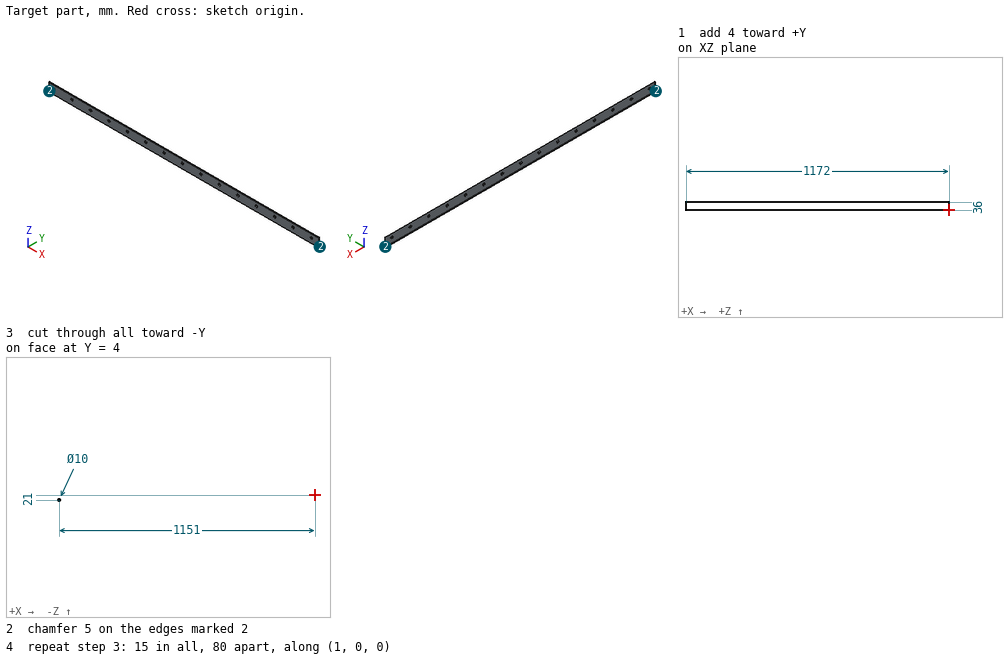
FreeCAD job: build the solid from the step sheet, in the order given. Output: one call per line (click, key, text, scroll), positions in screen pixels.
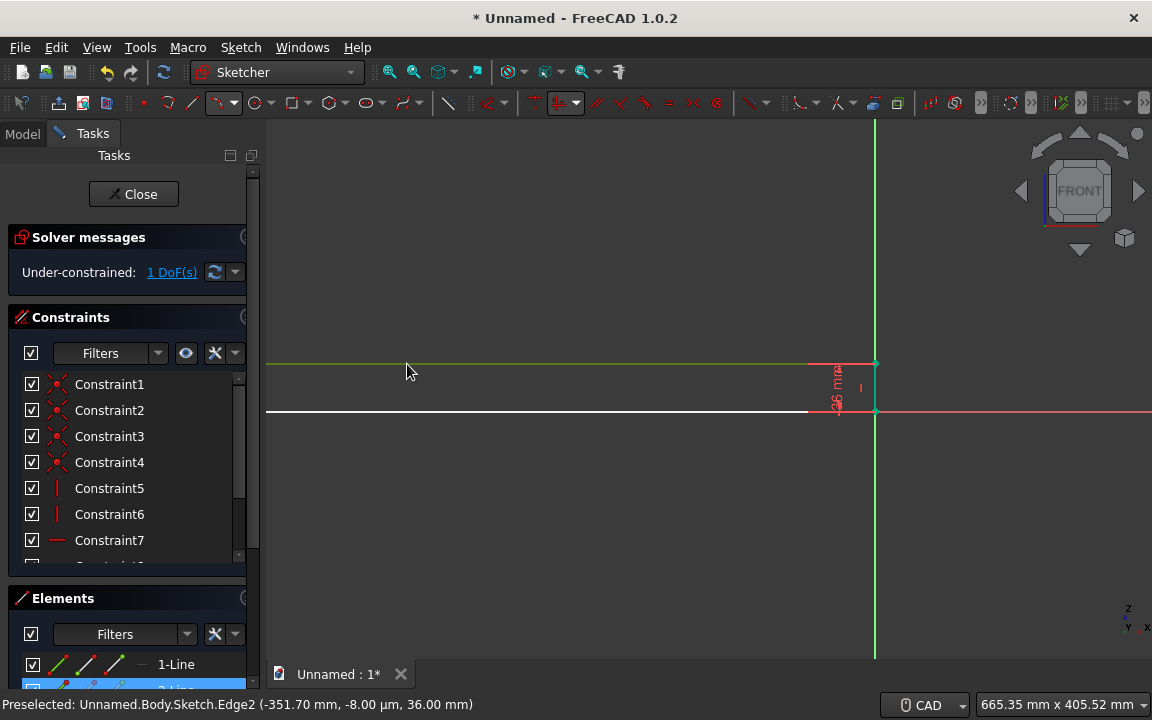
click(506, 104)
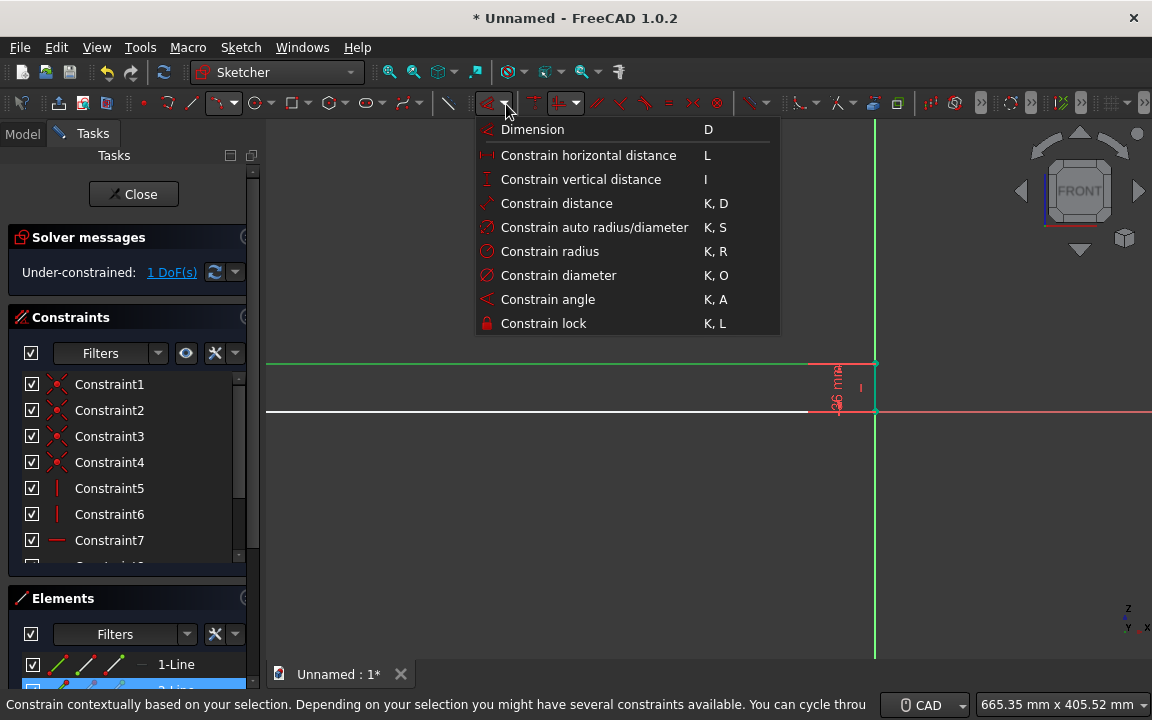
click(628, 155)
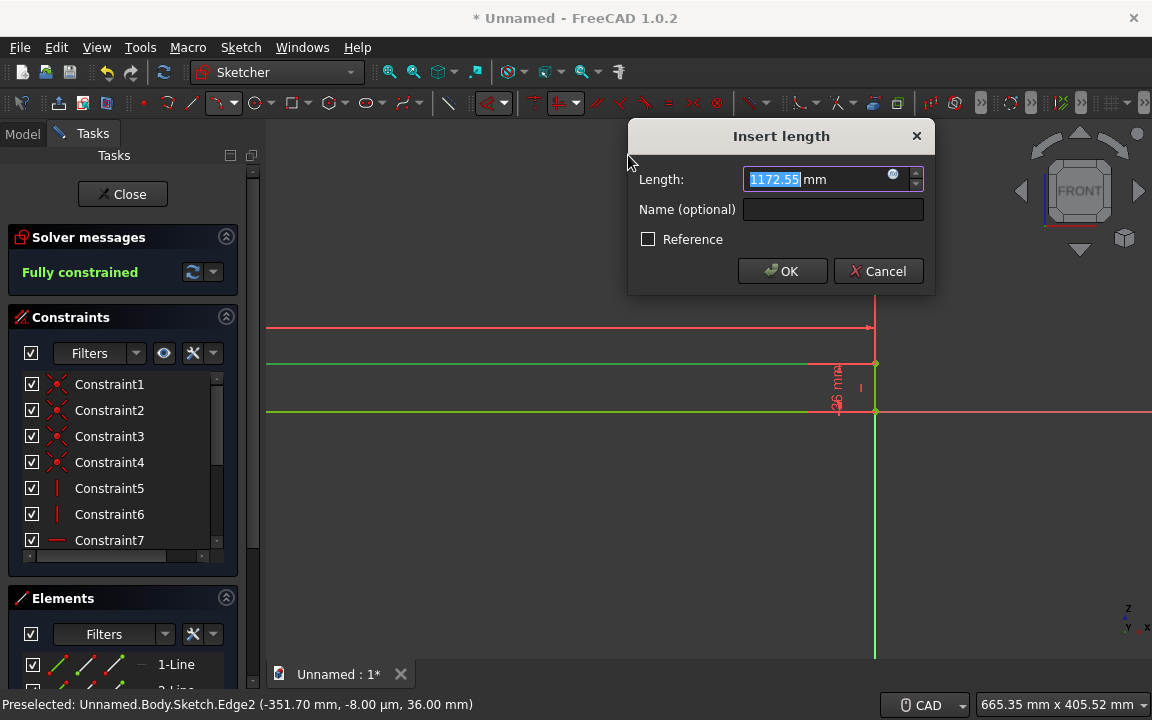
text(1172)
key(Return)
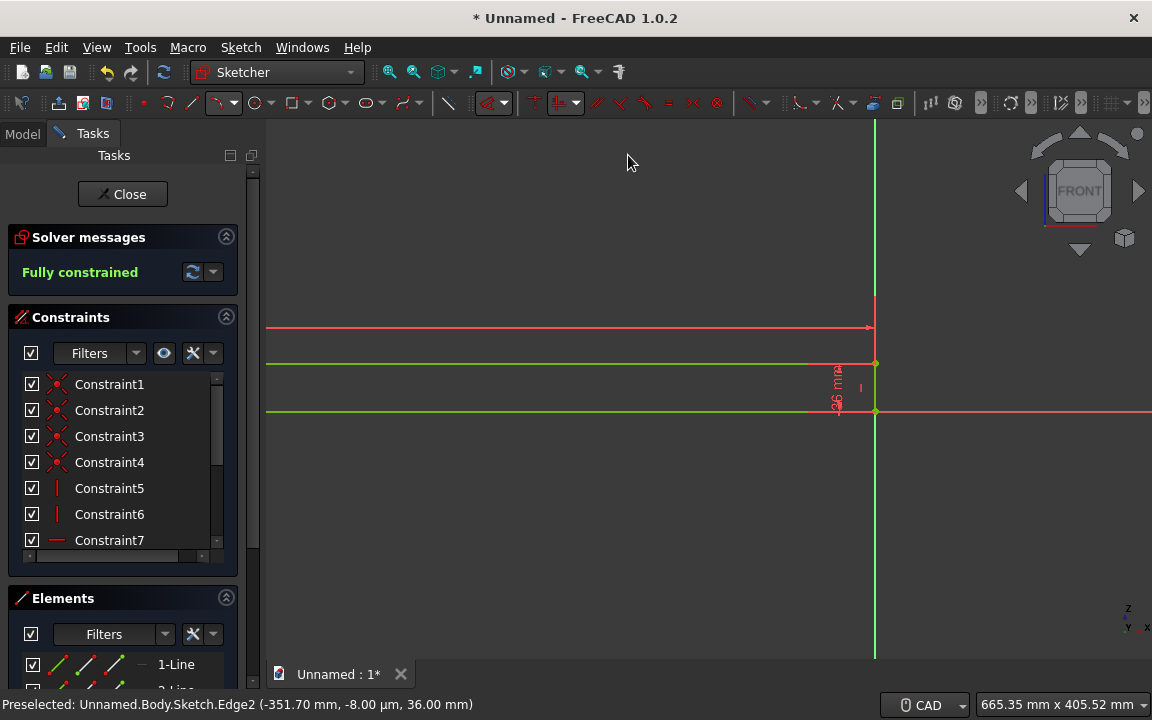
click(123, 194)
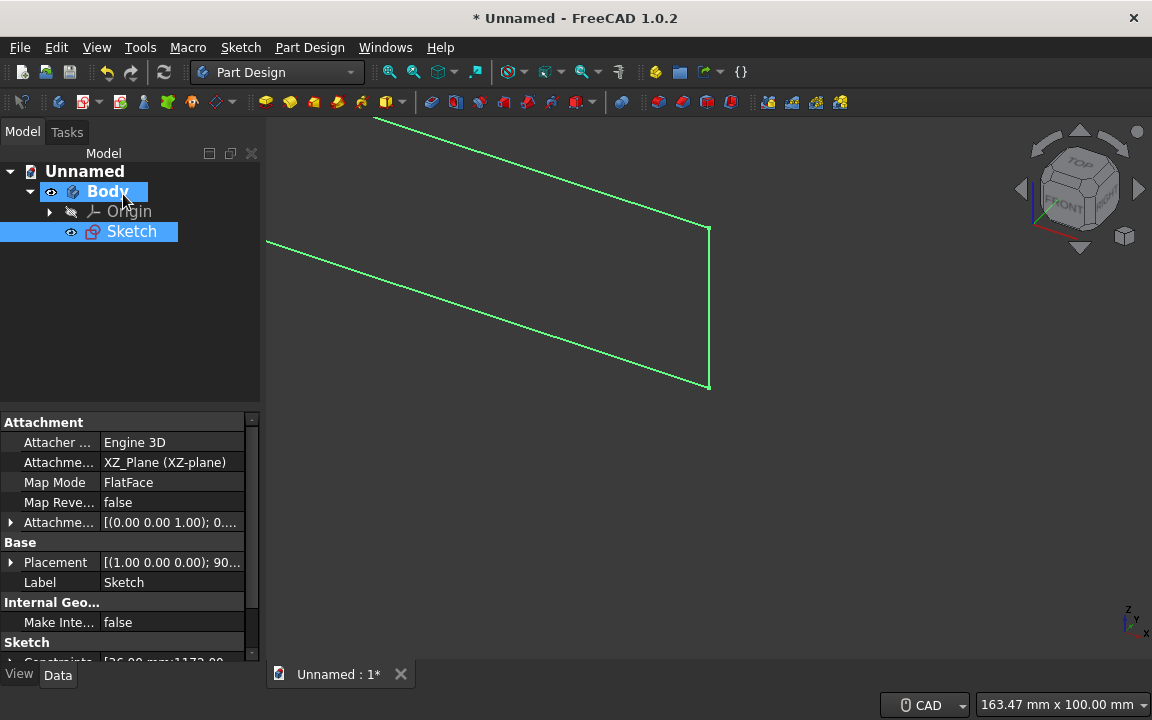
click(266, 102)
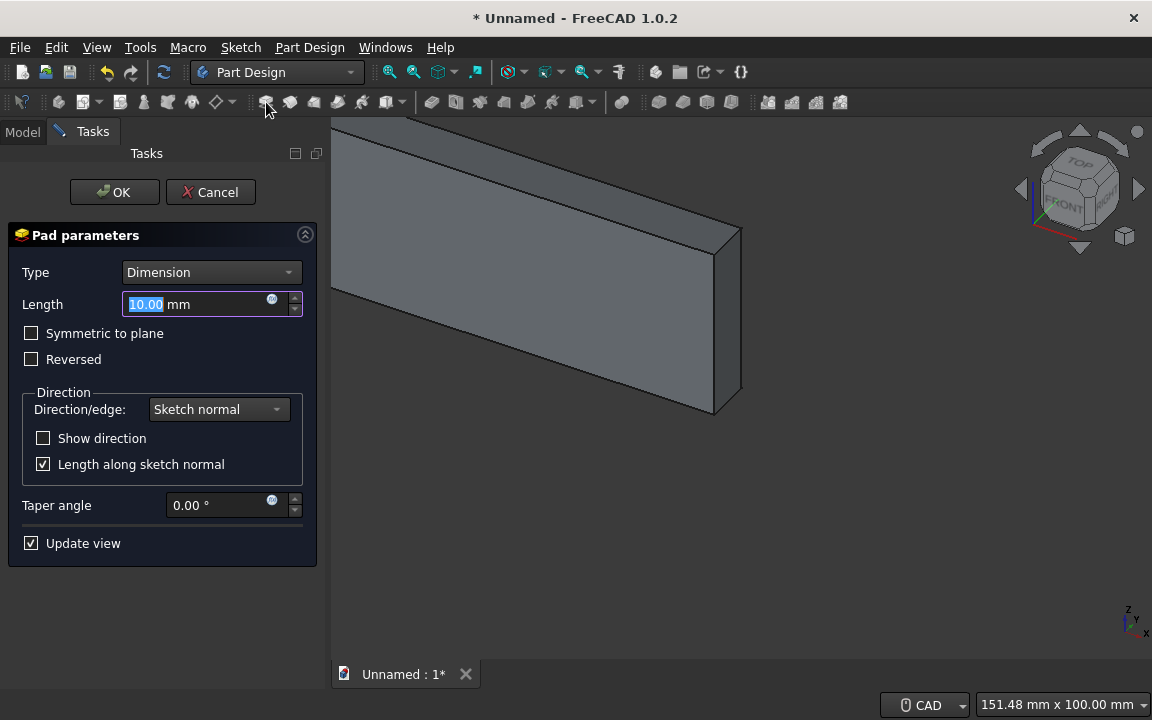
text(4)
key(Tab)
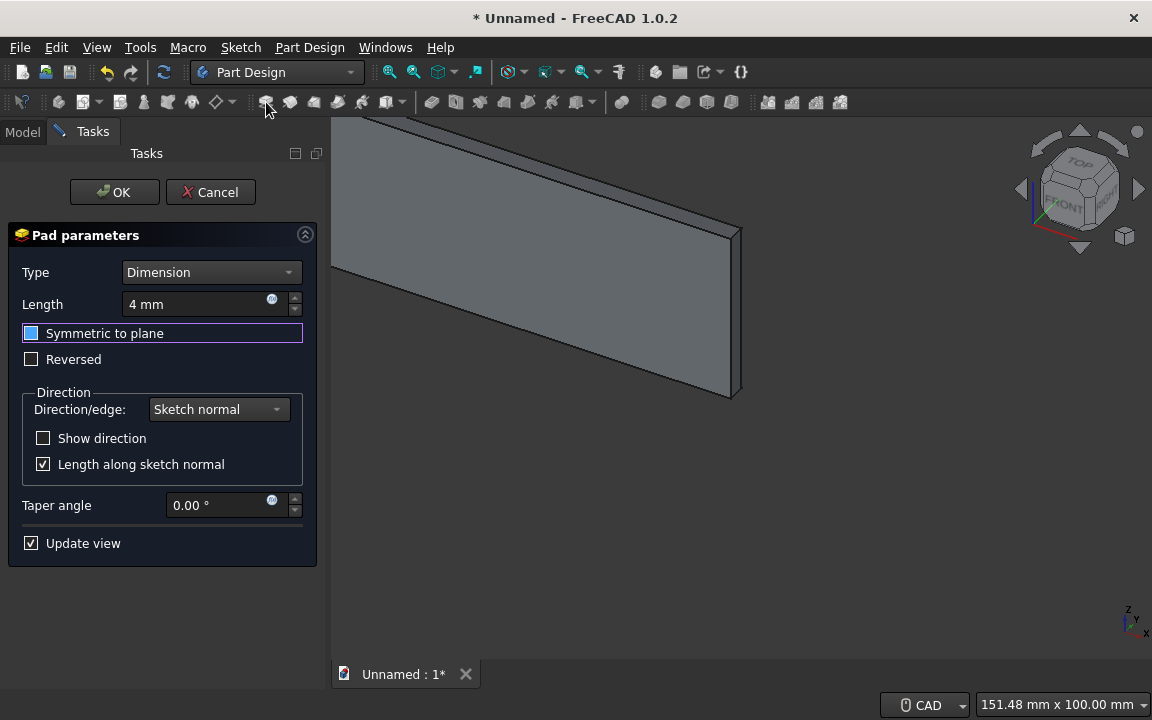
click(30, 359)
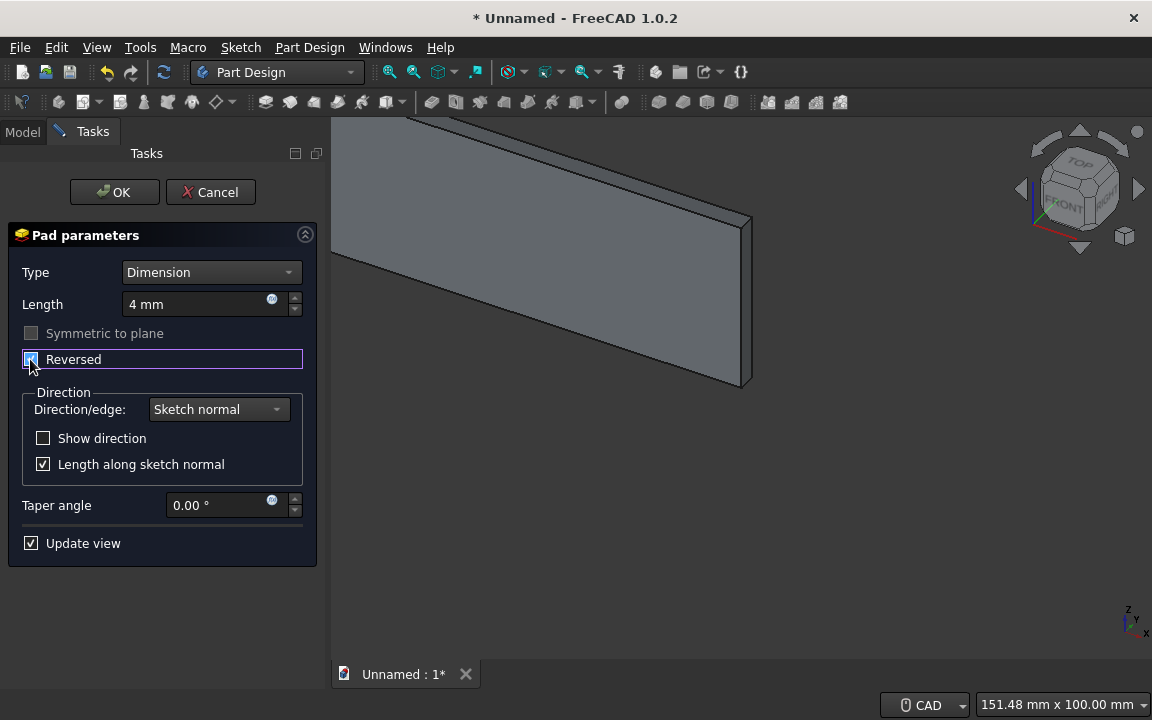
click(115, 192)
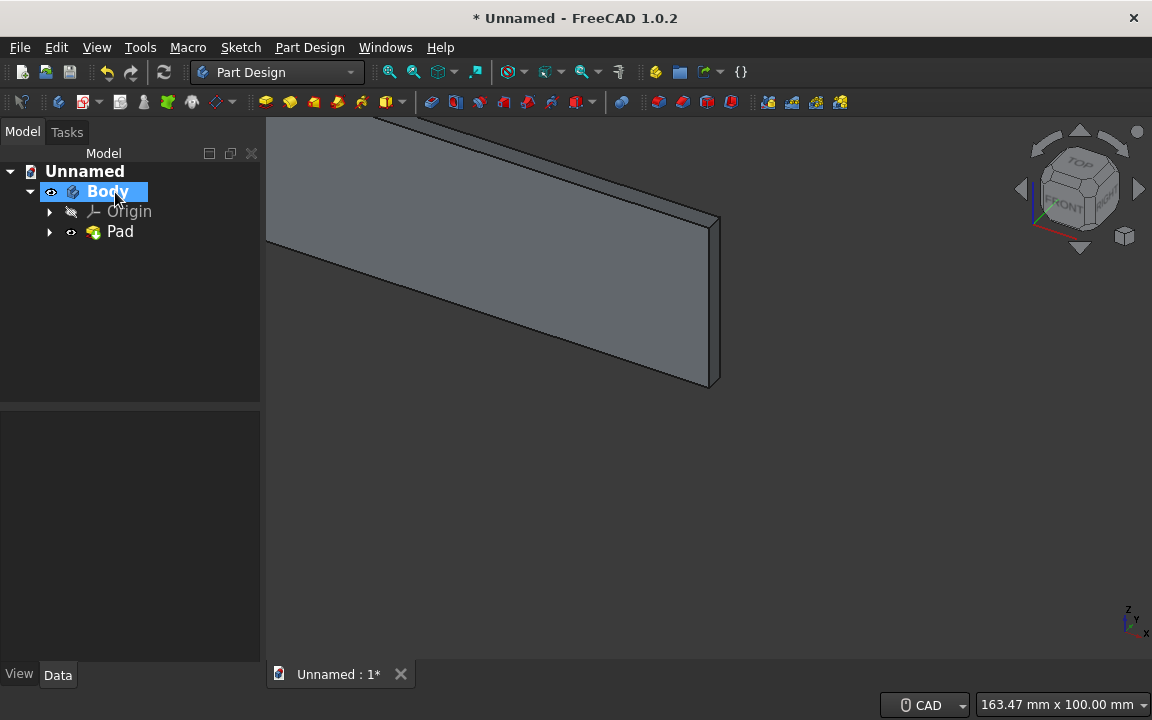
click(390, 72)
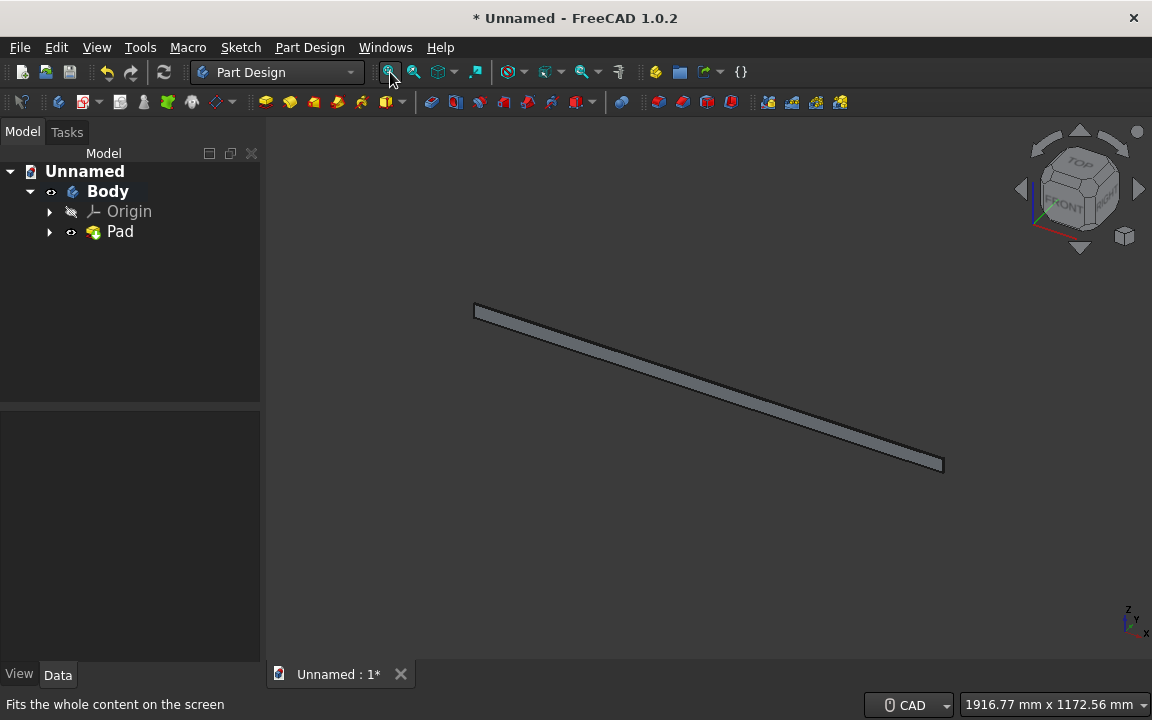
scroll(474, 316, up, 15)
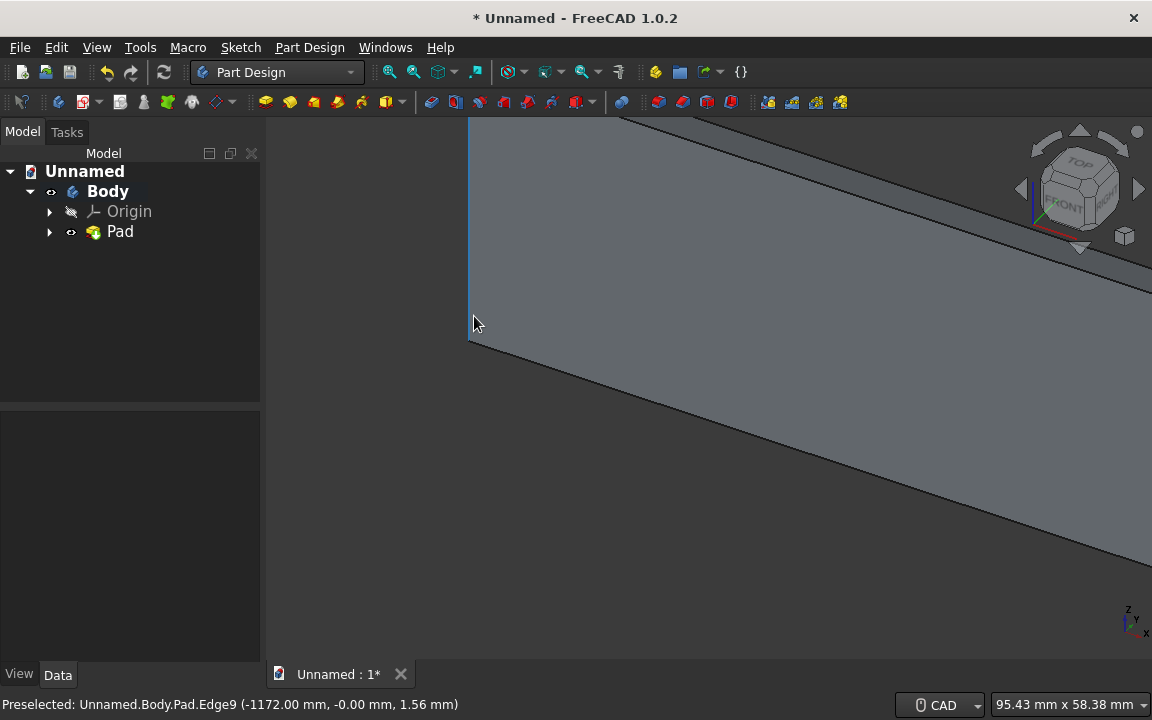
key(v)
key(f)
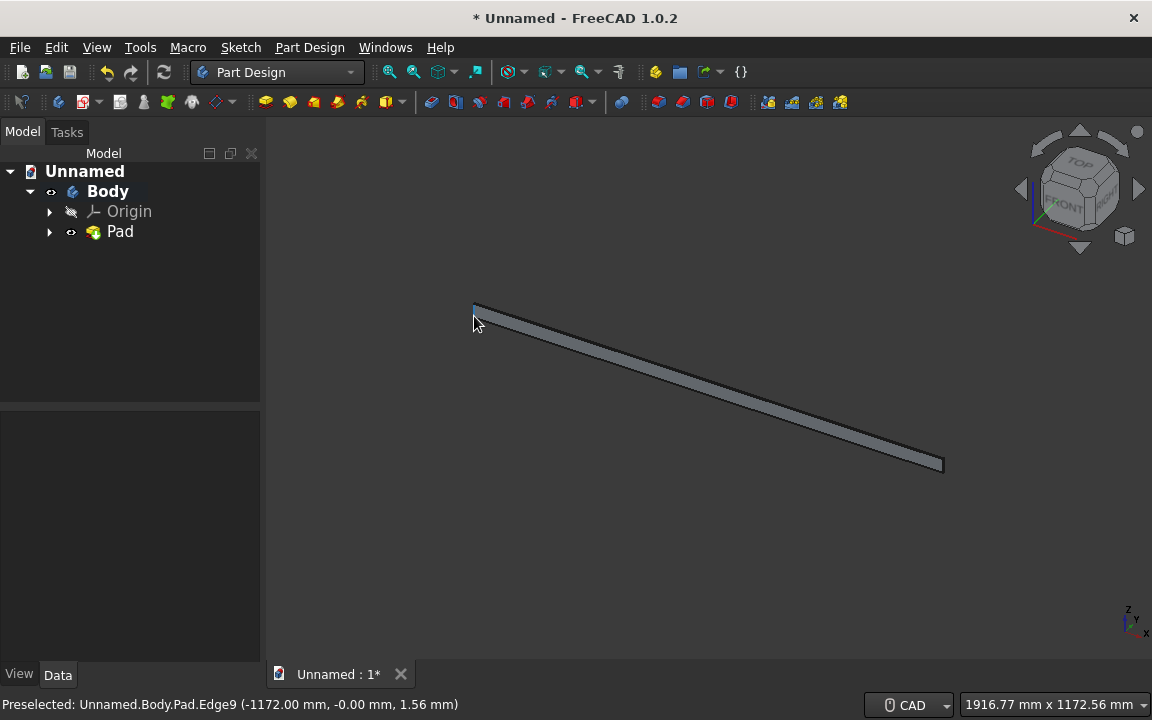
key(0)